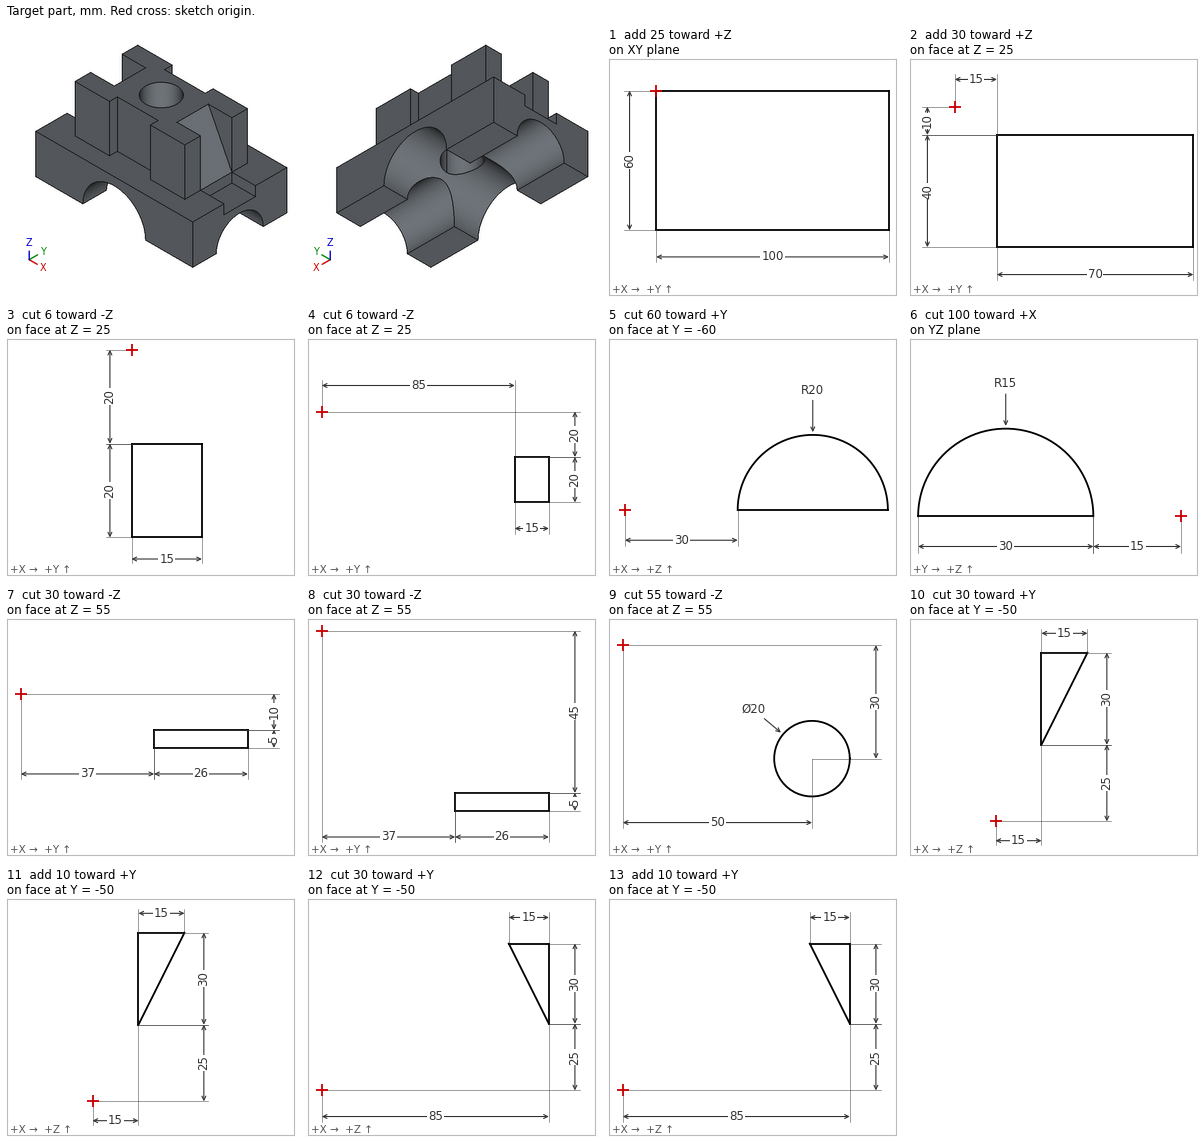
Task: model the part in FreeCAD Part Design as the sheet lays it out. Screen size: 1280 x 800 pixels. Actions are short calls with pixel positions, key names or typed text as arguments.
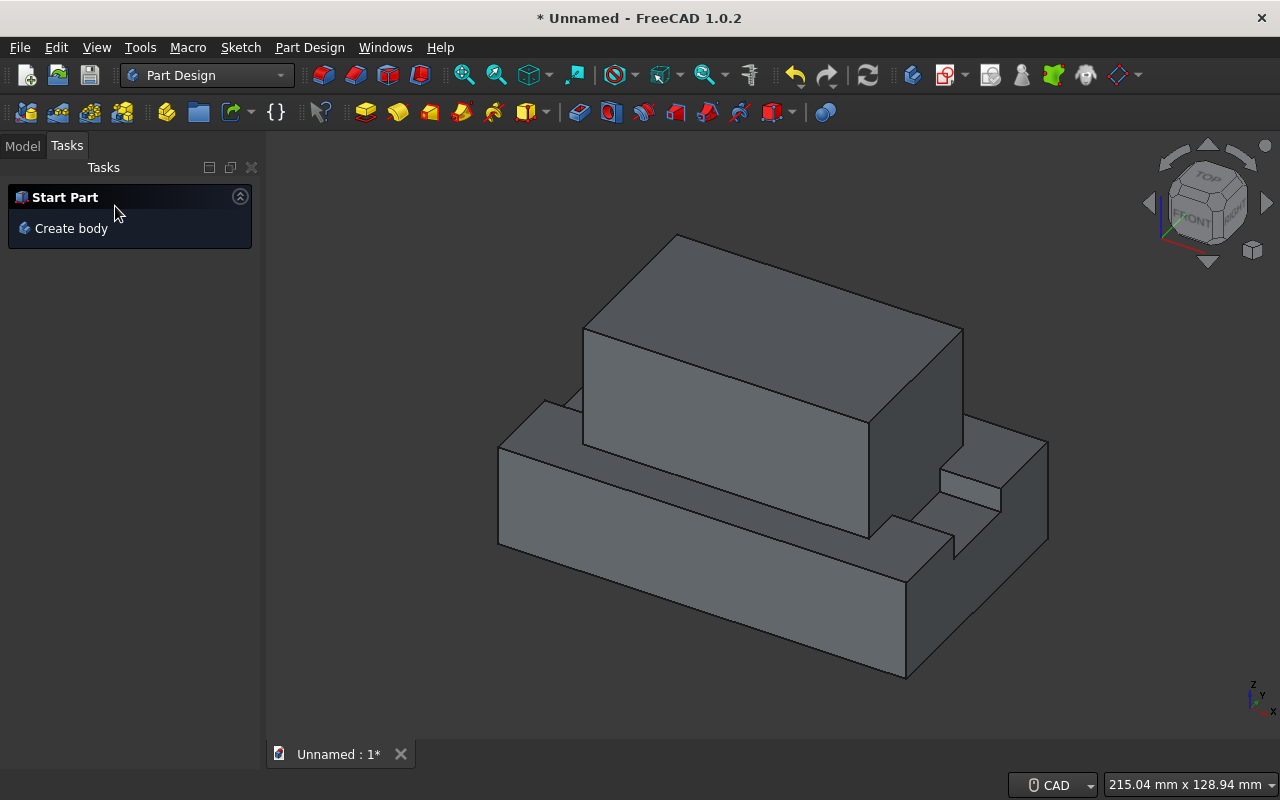
click(819, 601)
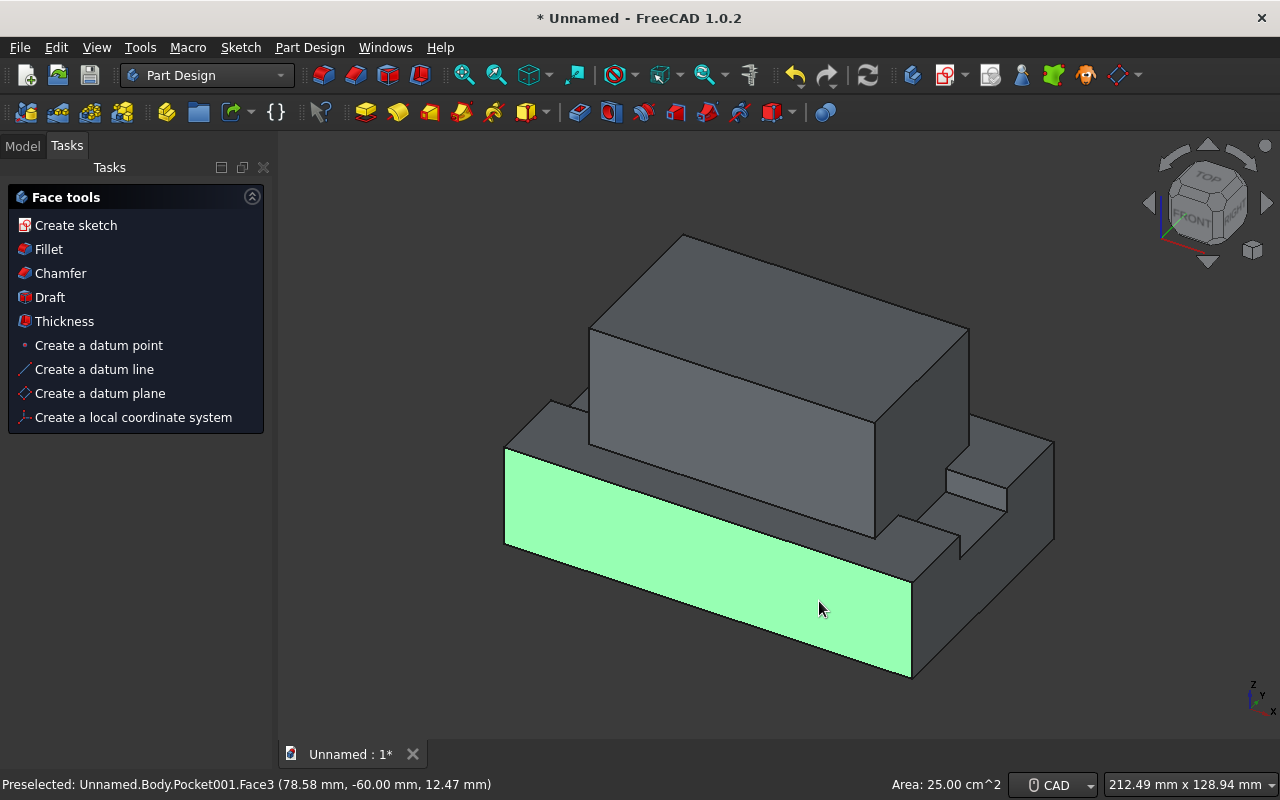
click(946, 76)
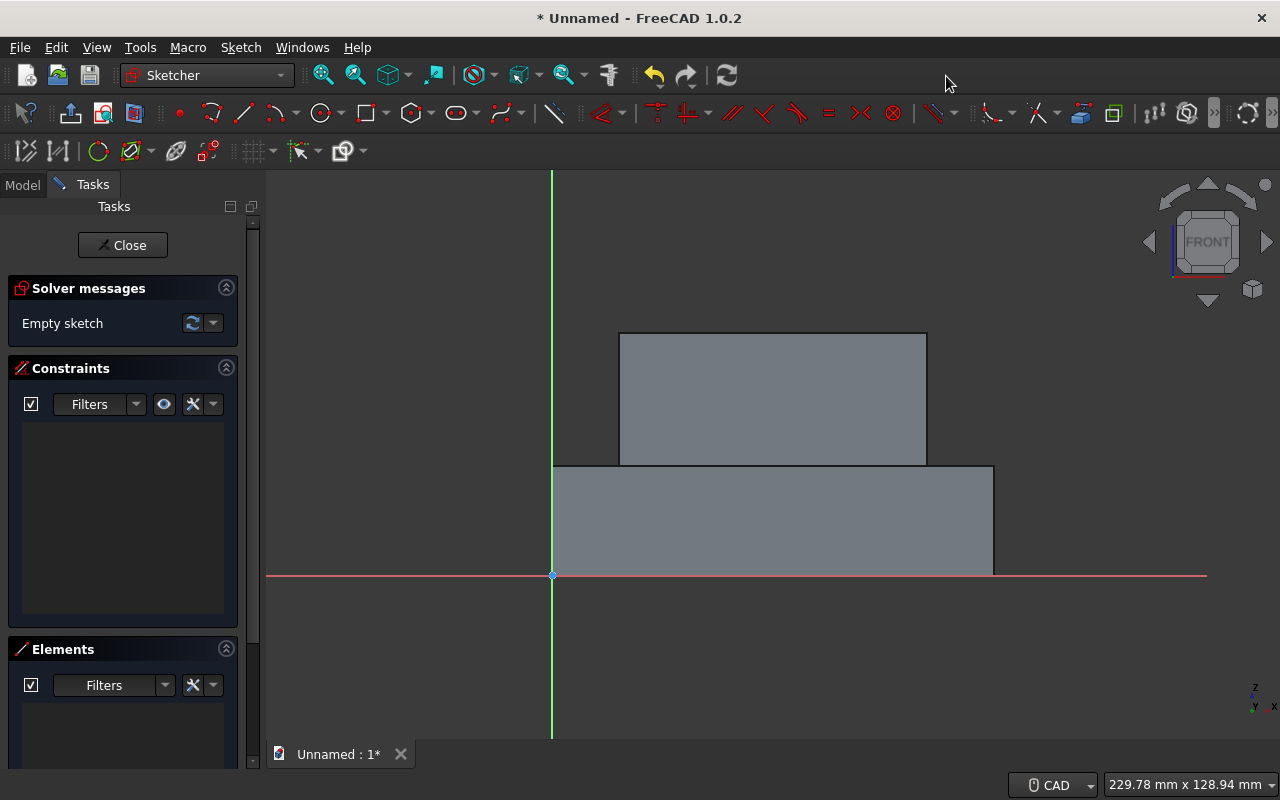
scroll(710, 626, up, 3)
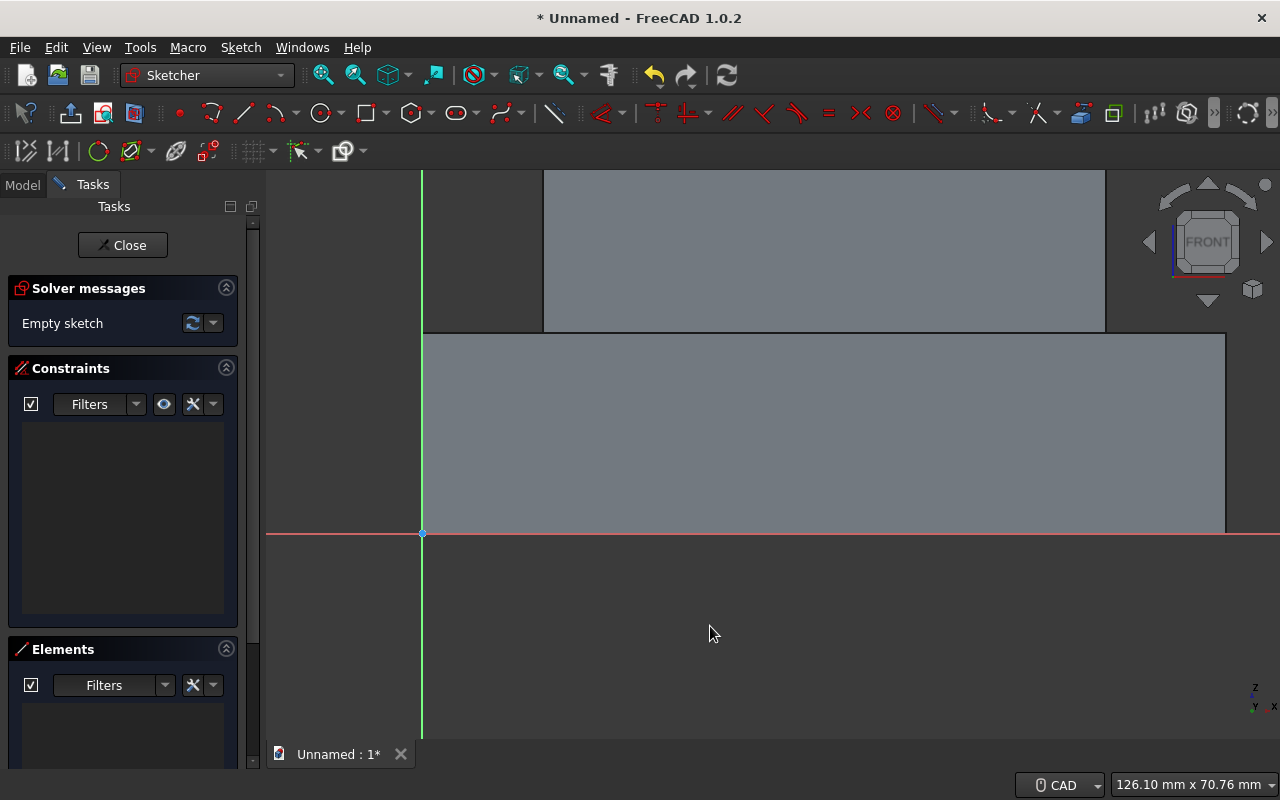
click(244, 114)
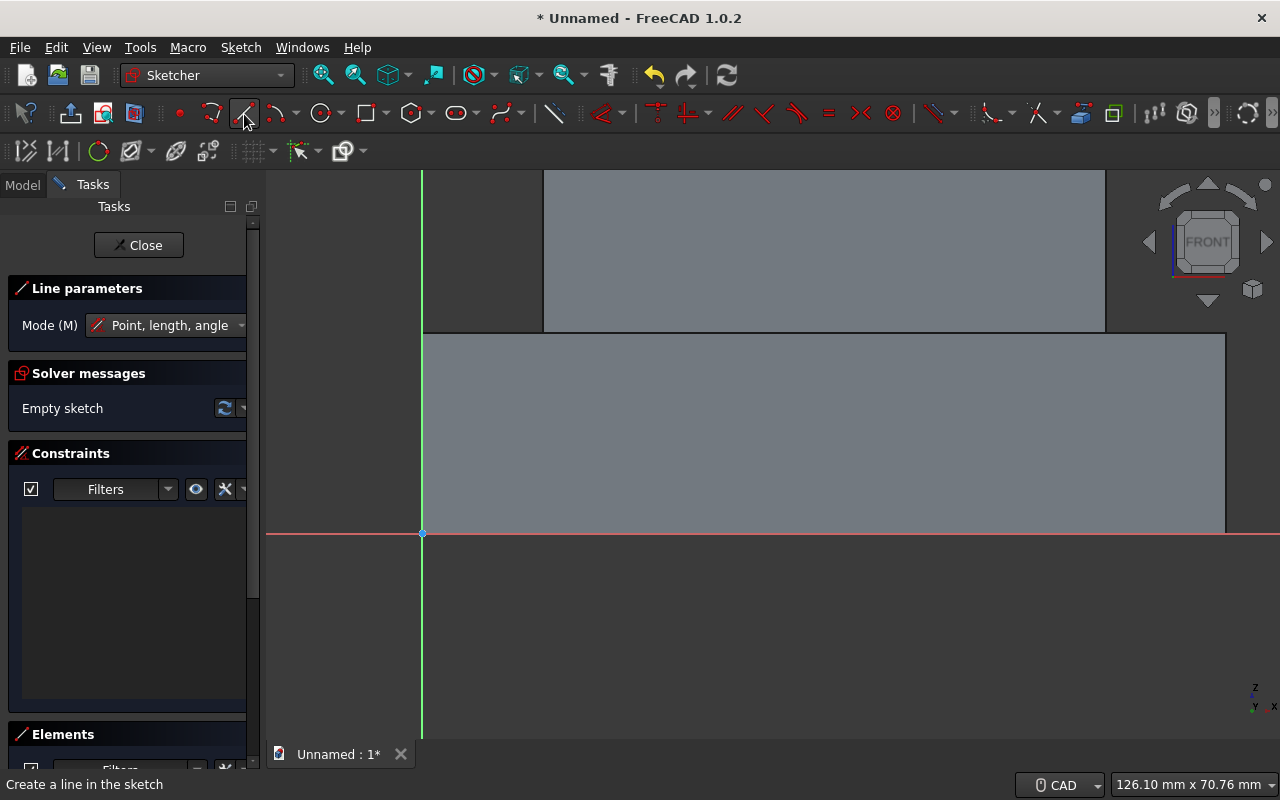
click(664, 534)
click(985, 525)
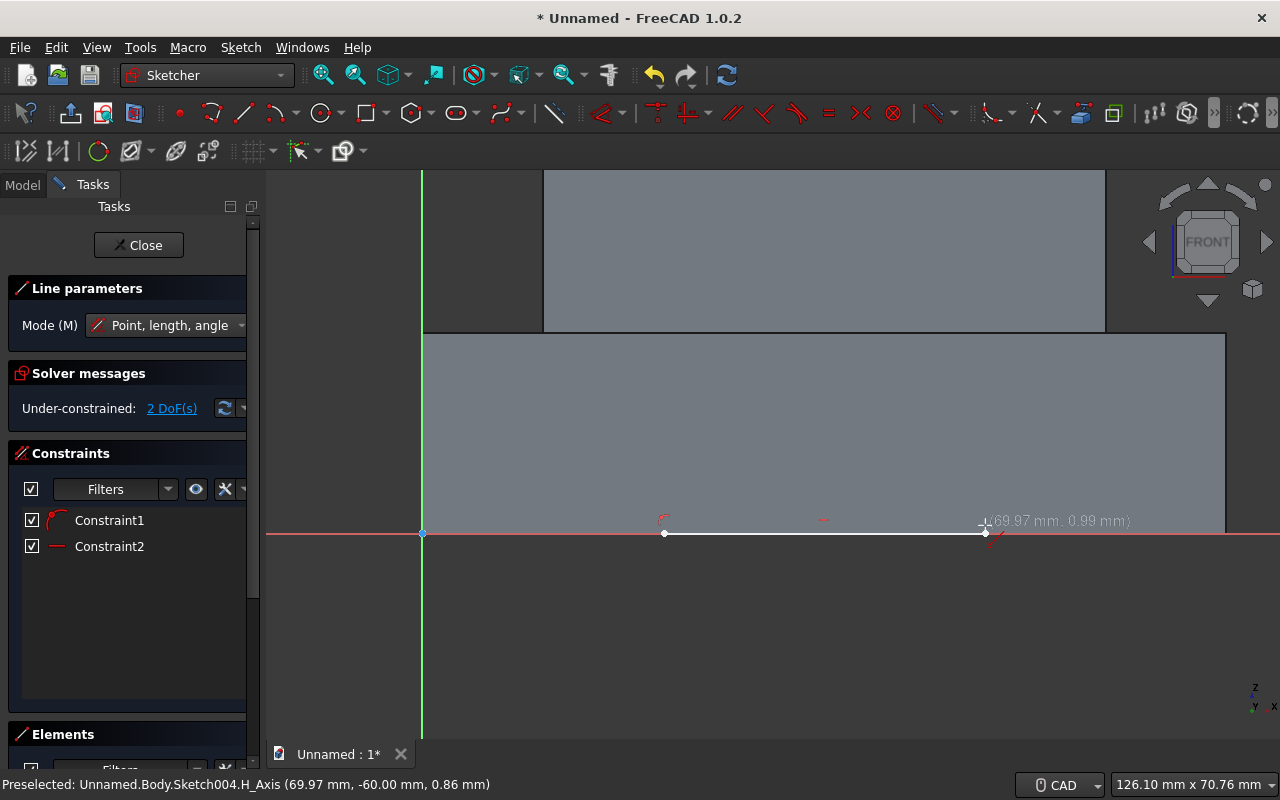
key(g)
key(3)
key(a)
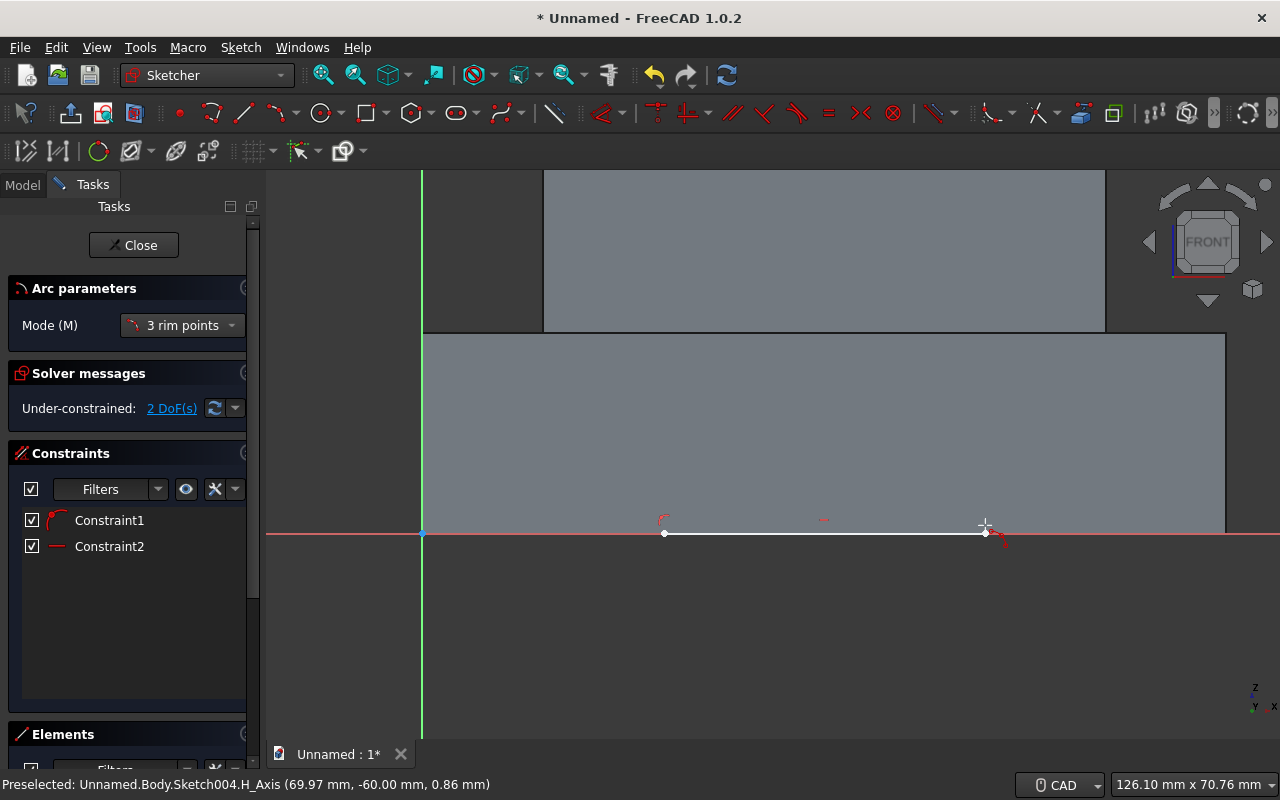
click(985, 534)
click(664, 534)
click(824, 373)
key(Escape)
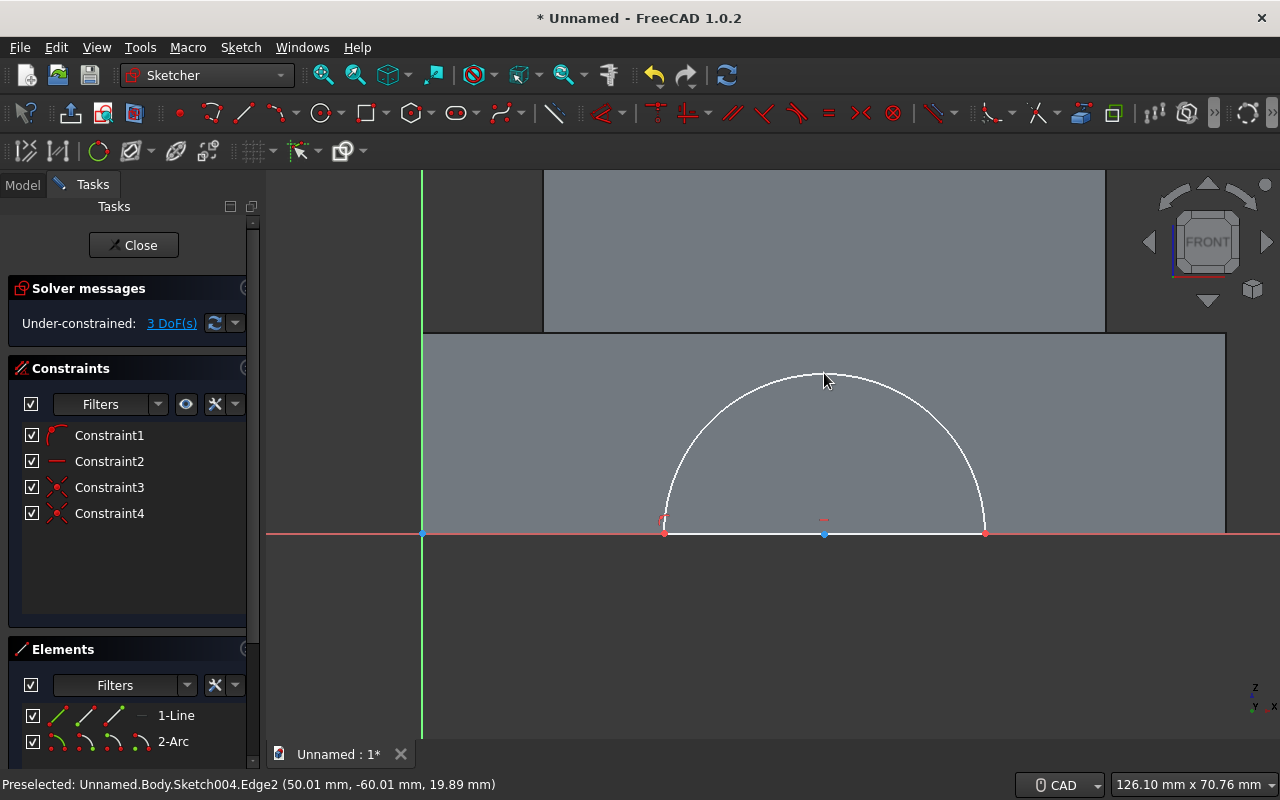
click(825, 535)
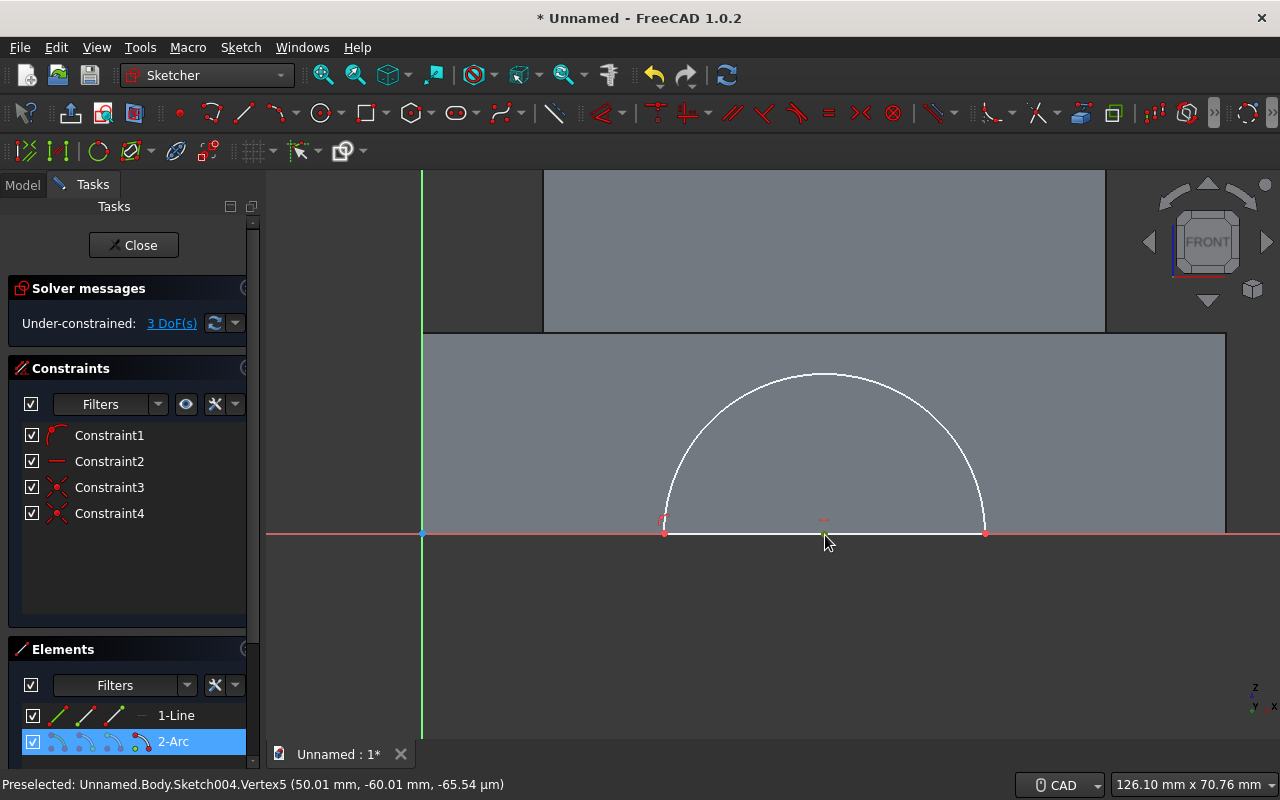
click(353, 534)